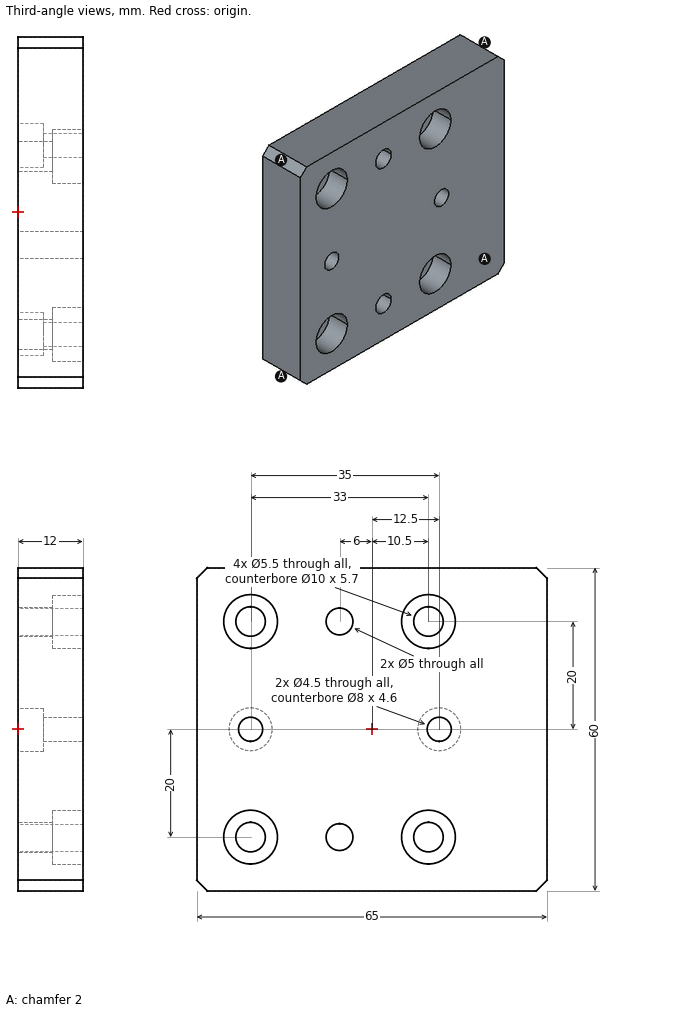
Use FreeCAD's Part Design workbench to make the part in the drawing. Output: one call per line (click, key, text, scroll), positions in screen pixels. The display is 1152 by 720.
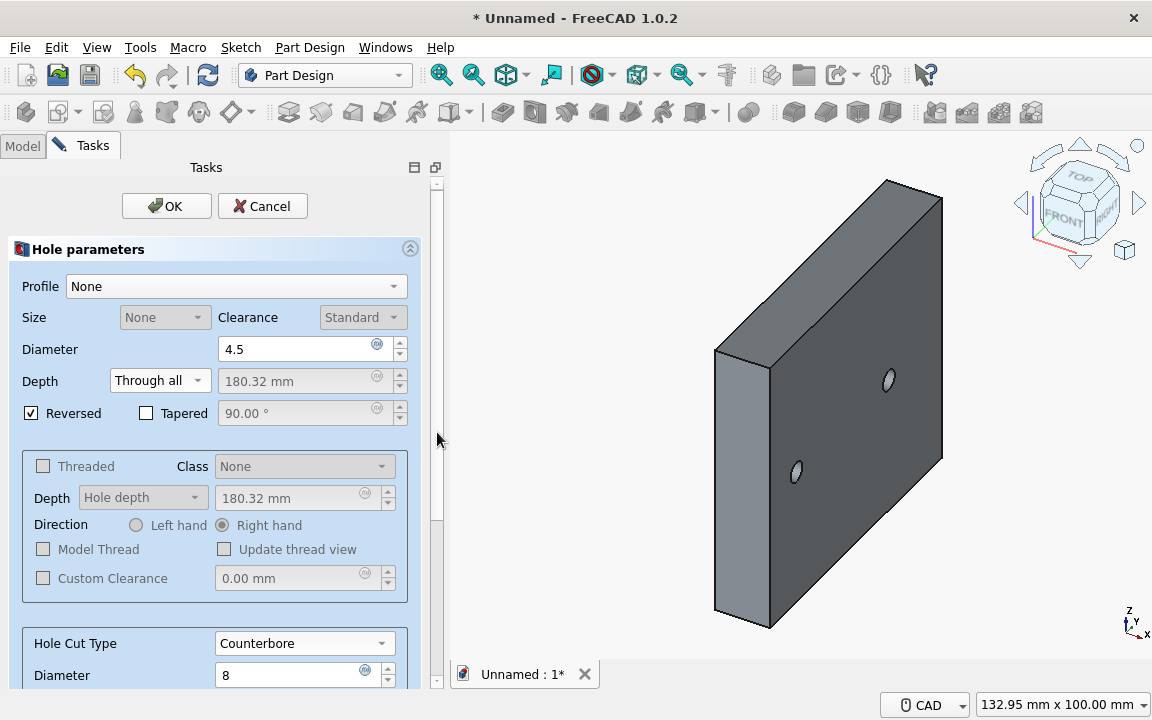
click(167, 206)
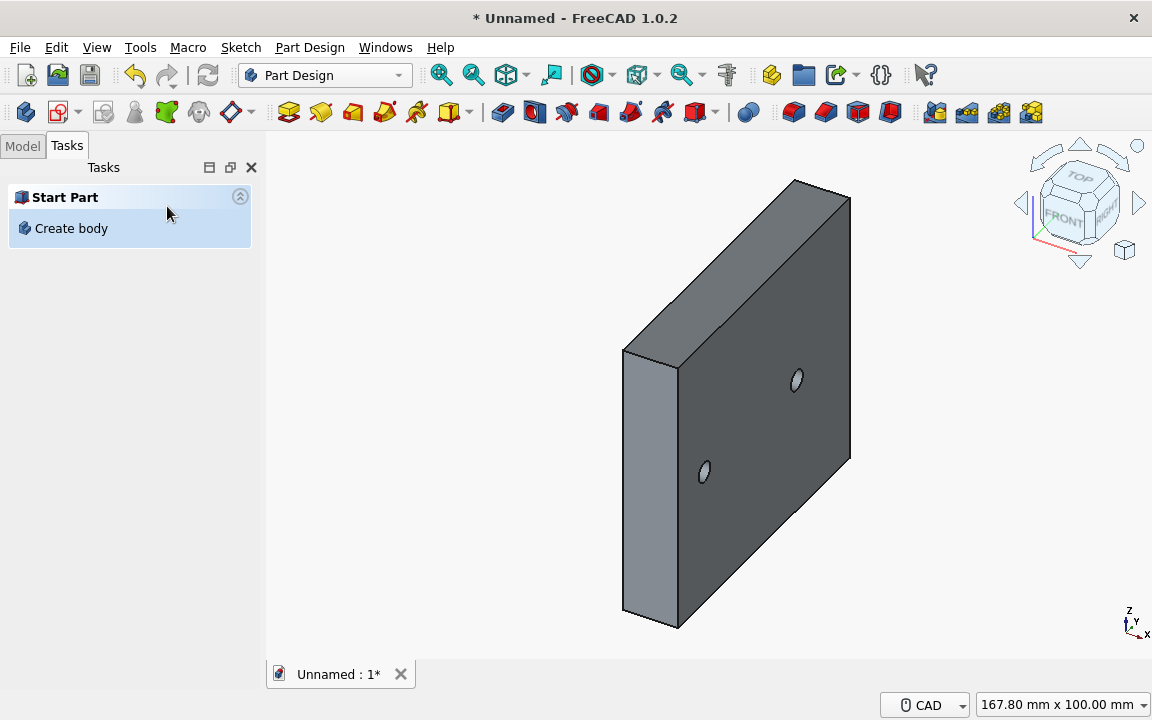
click(739, 474)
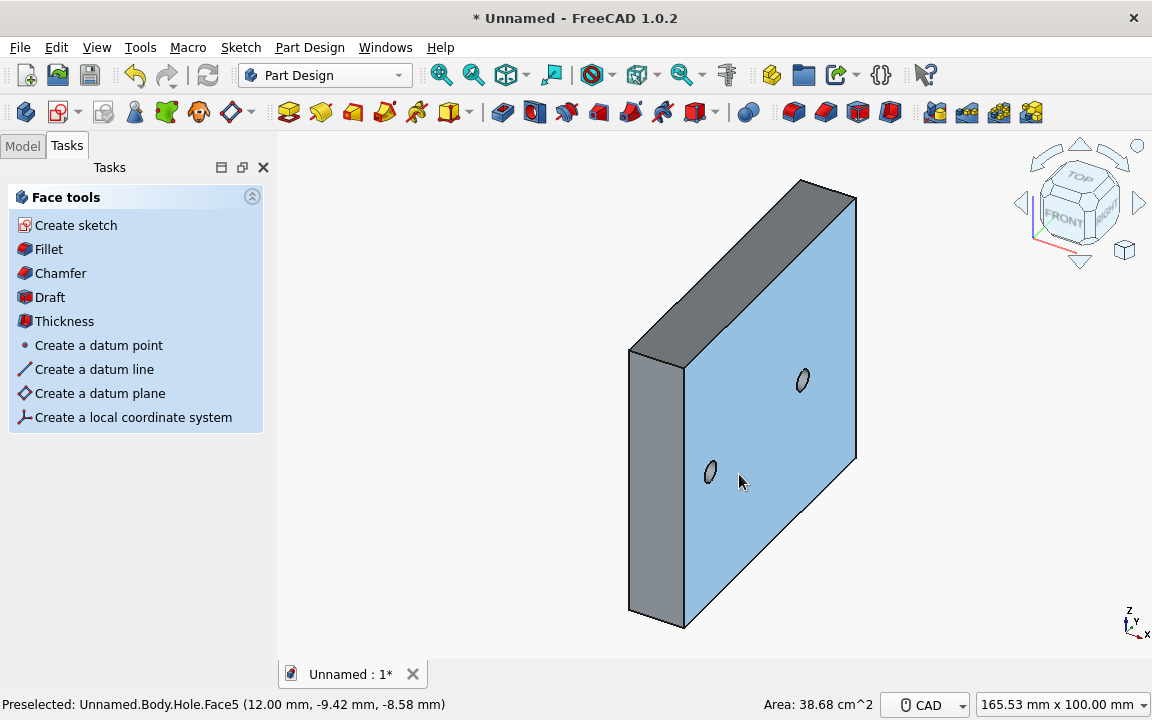
click(58, 112)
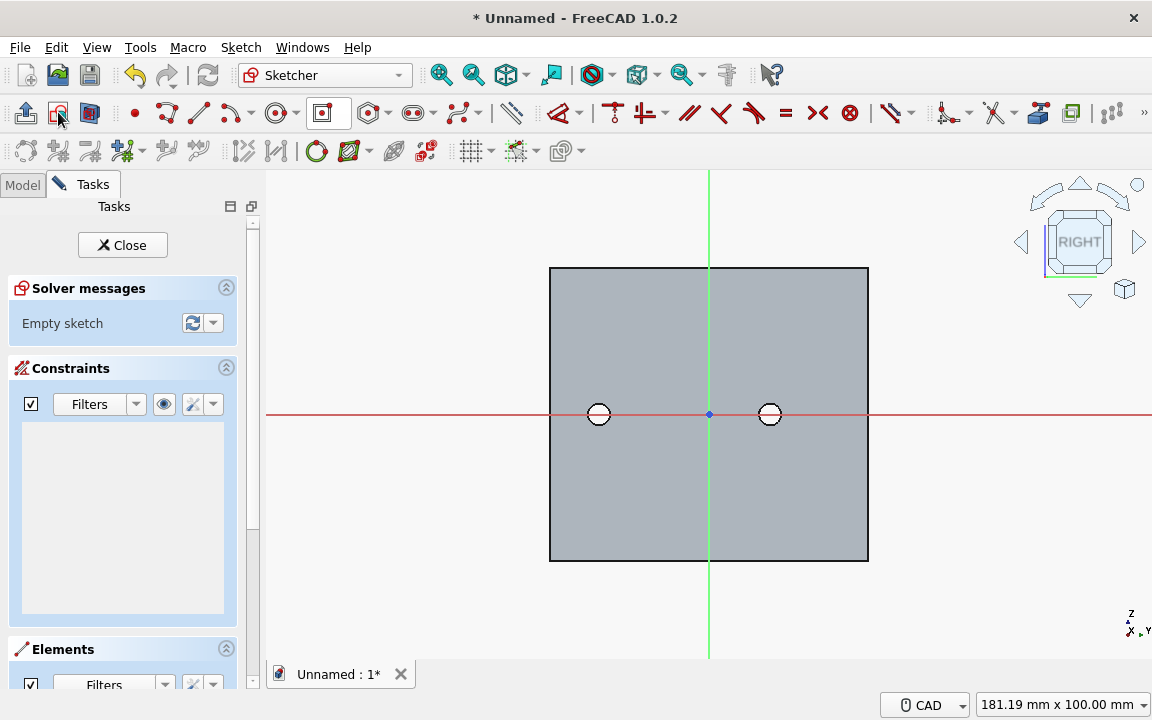
scroll(759, 414, up, 2)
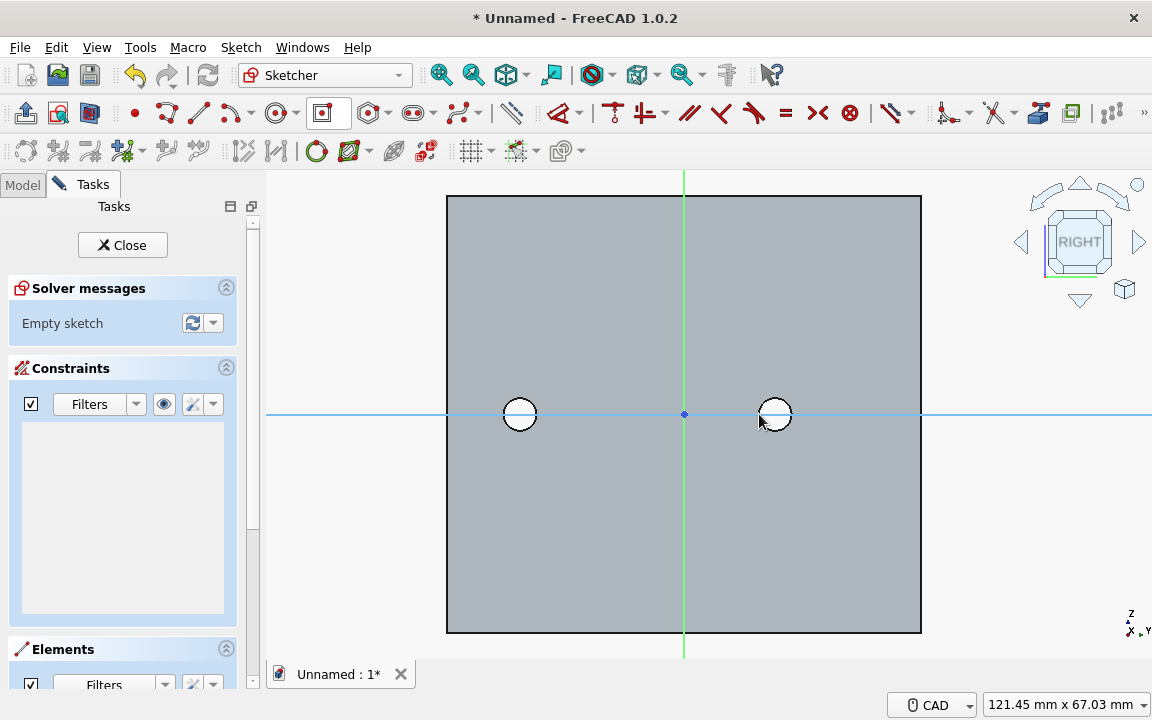
click(276, 114)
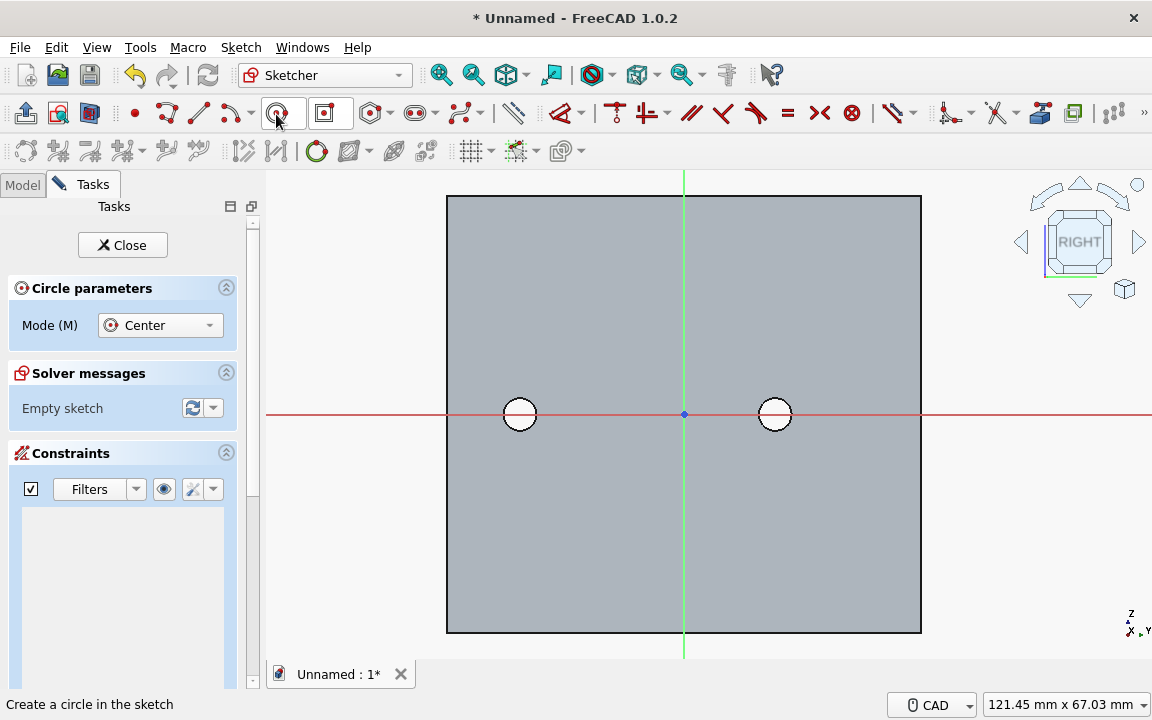
click(761, 269)
click(775, 254)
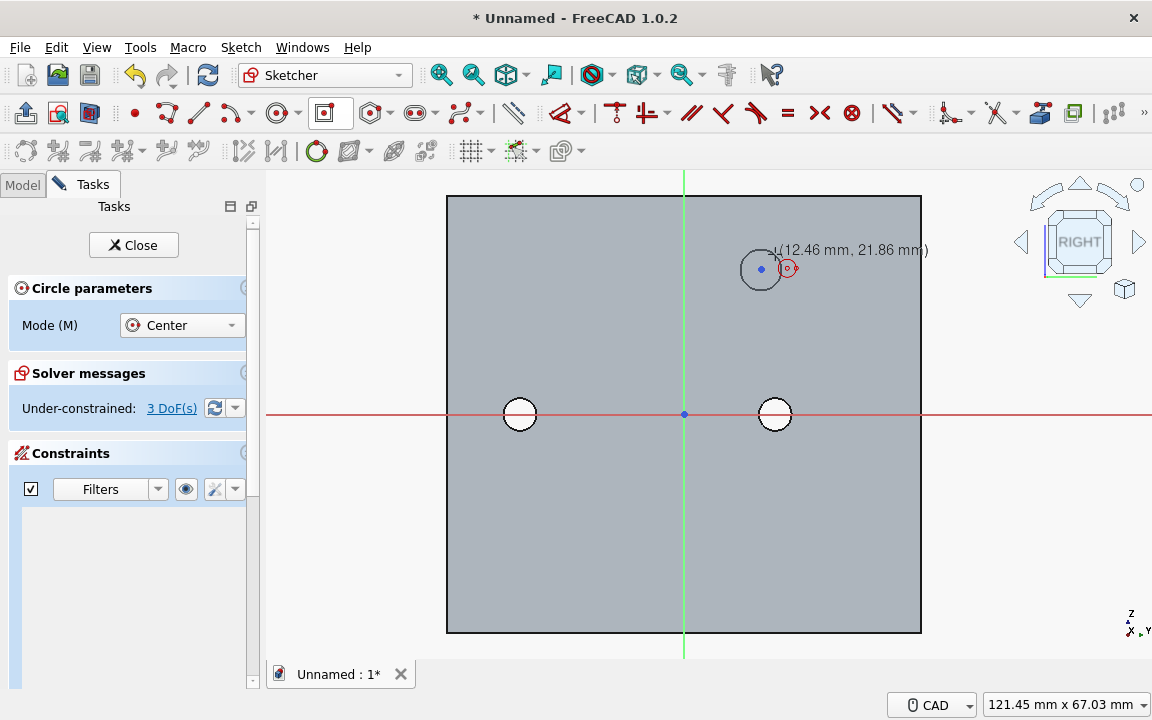
click(520, 269)
click(534, 254)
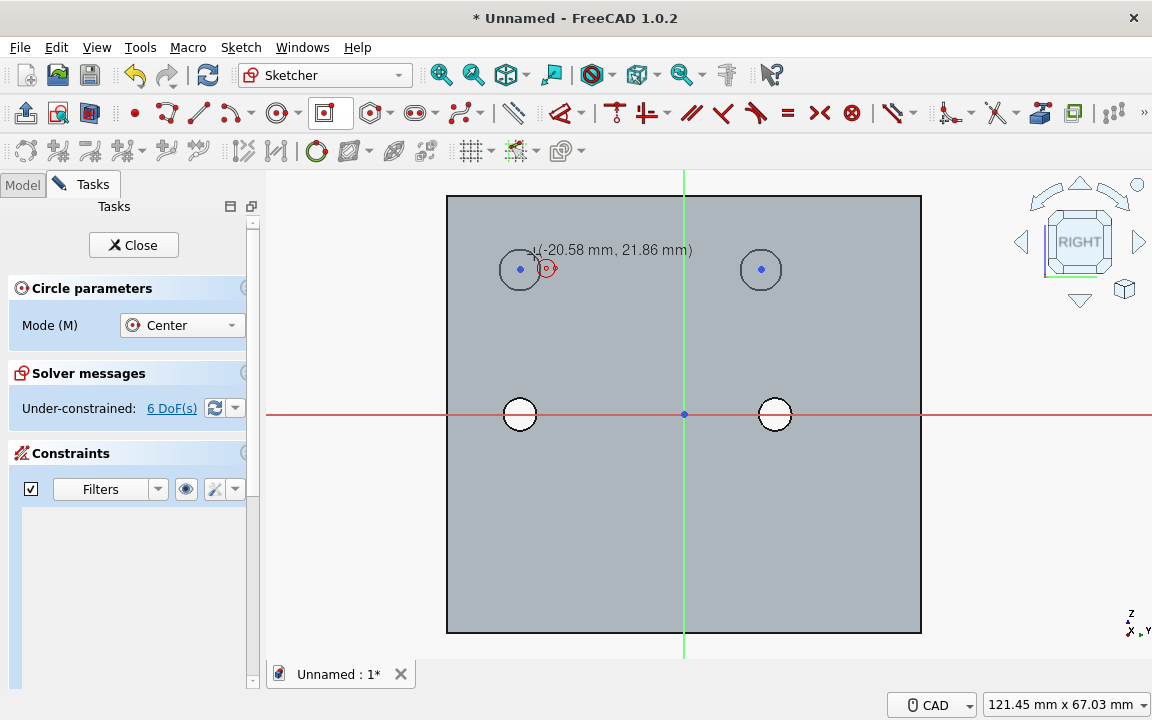
click(520, 560)
click(534, 546)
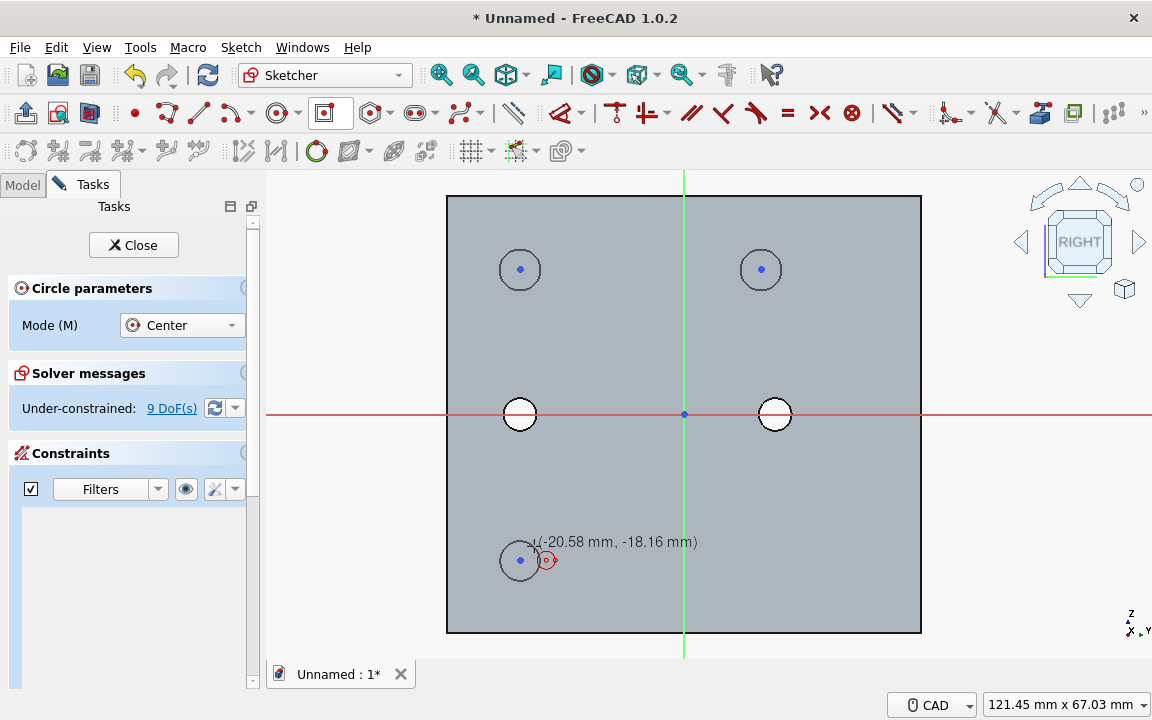
click(761, 560)
click(775, 546)
key(Escape)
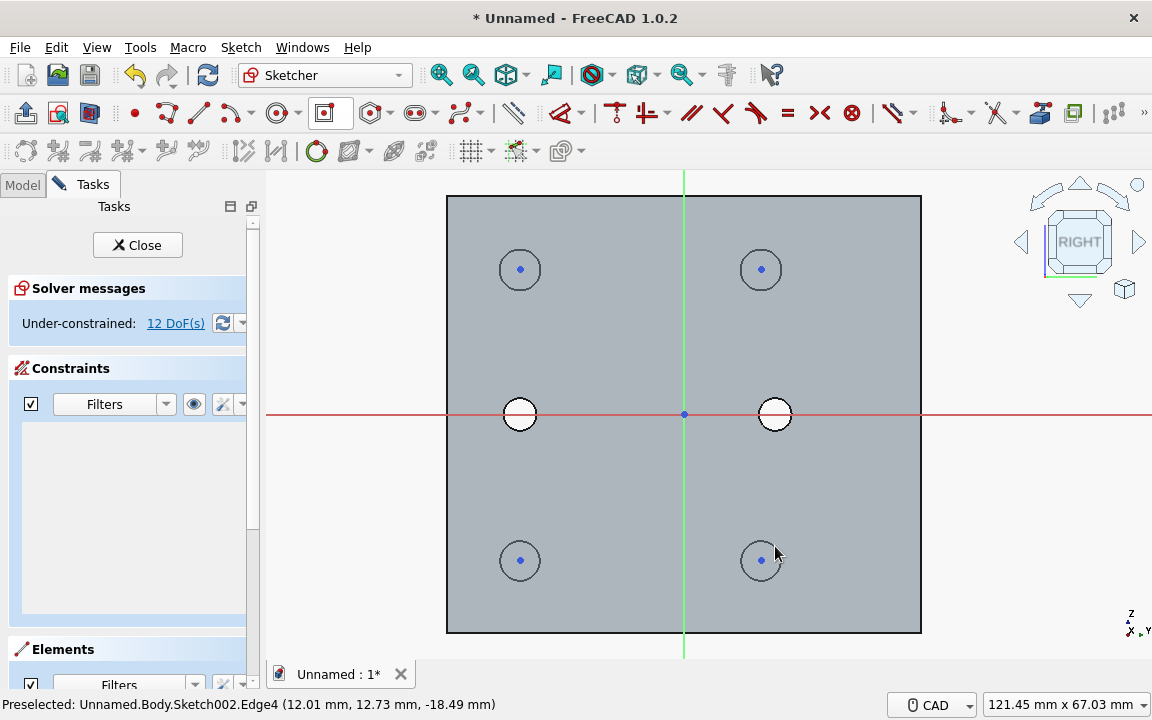
click(775, 255)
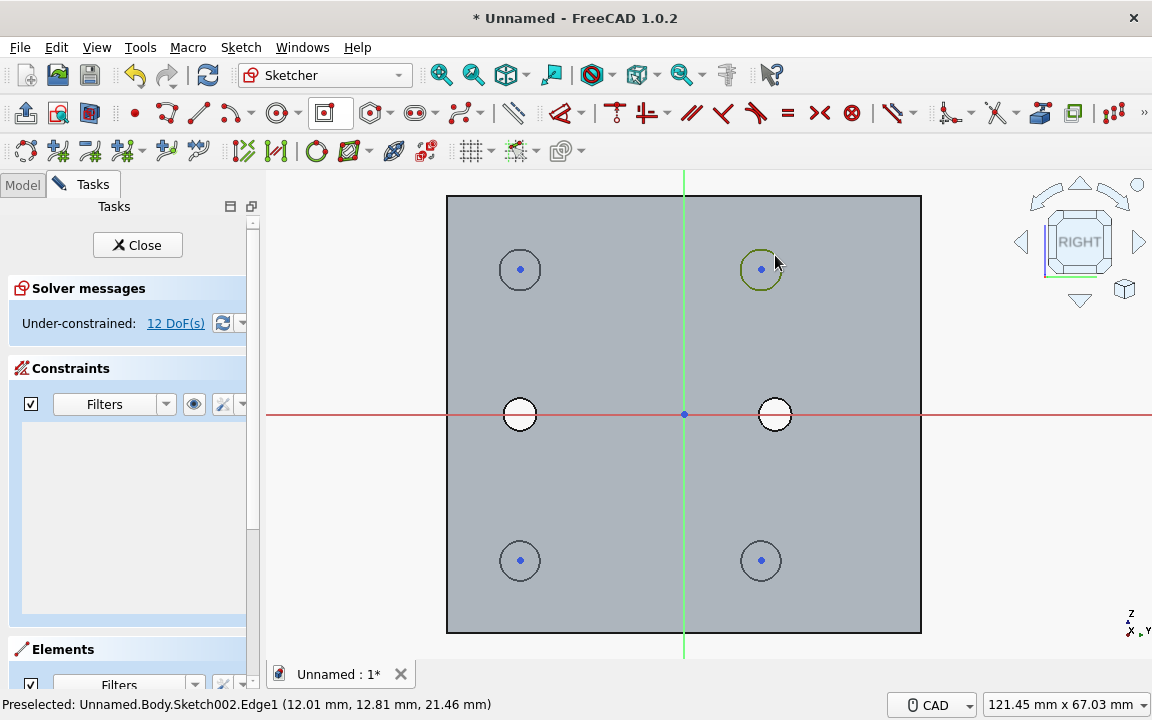
click(534, 255)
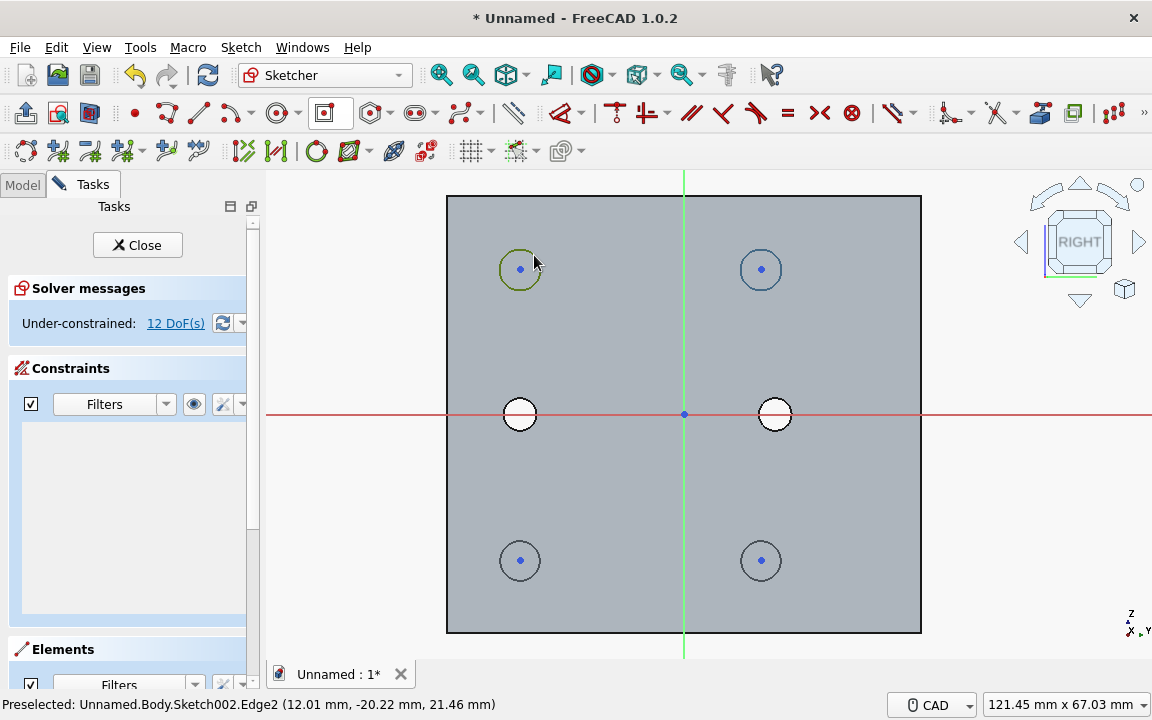
click(534, 547)